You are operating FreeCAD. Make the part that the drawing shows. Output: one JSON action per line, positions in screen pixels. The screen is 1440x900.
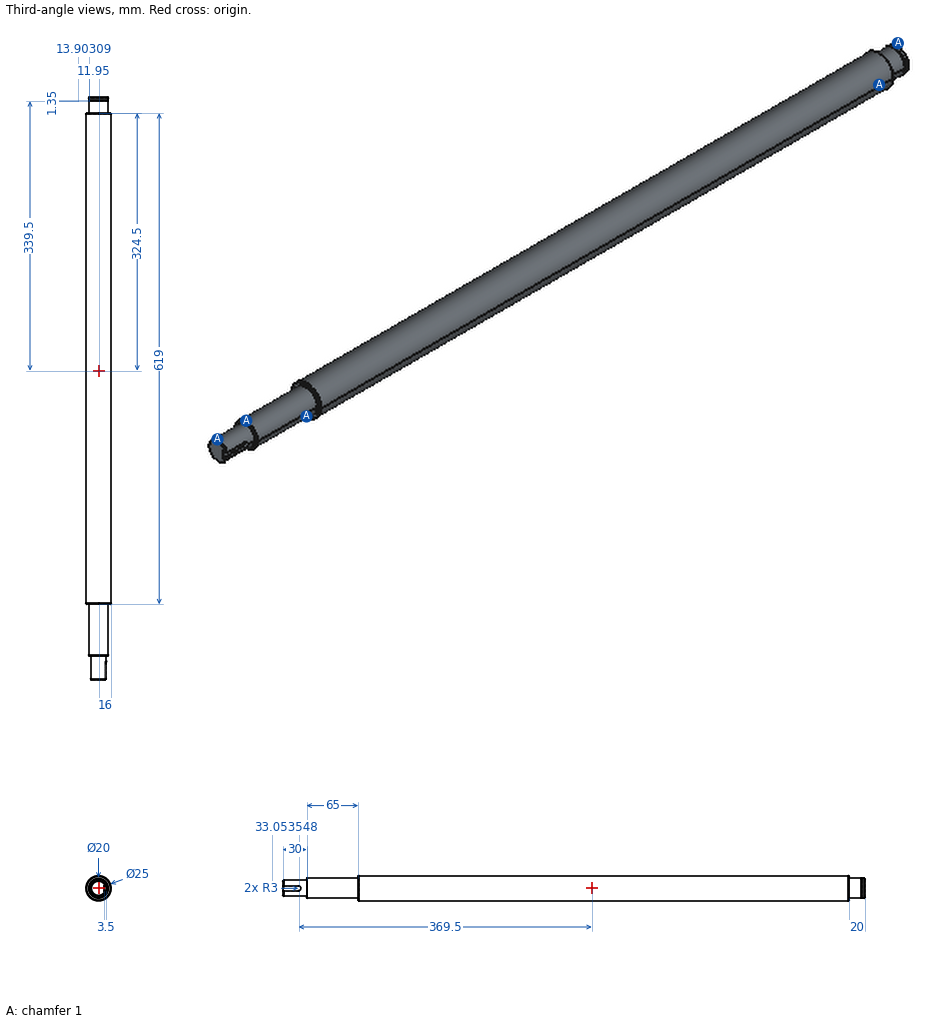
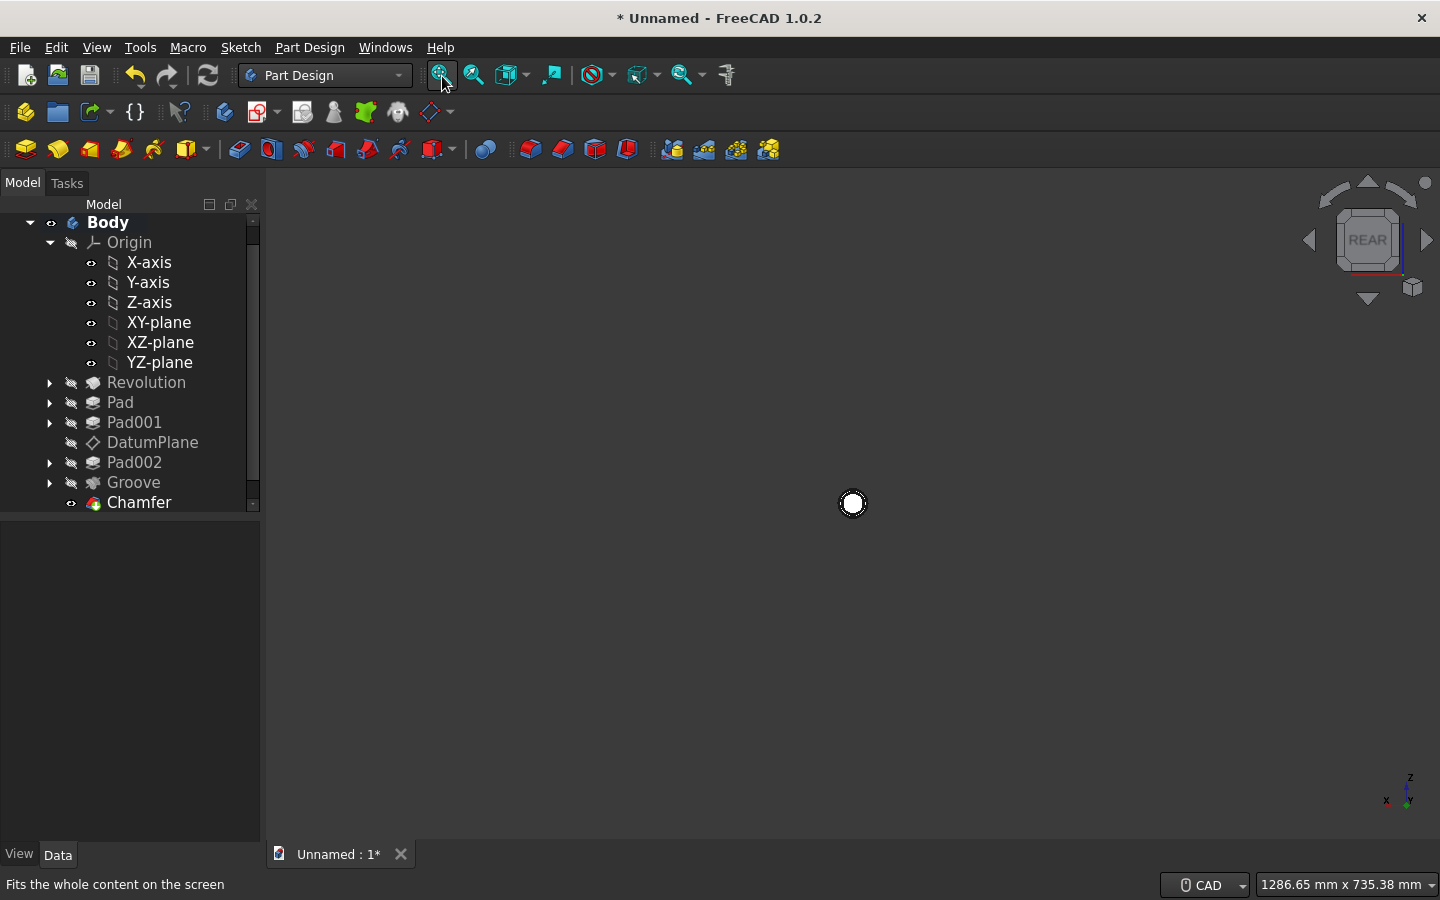
{"action": "left_click", "coordinate": [136, 363]}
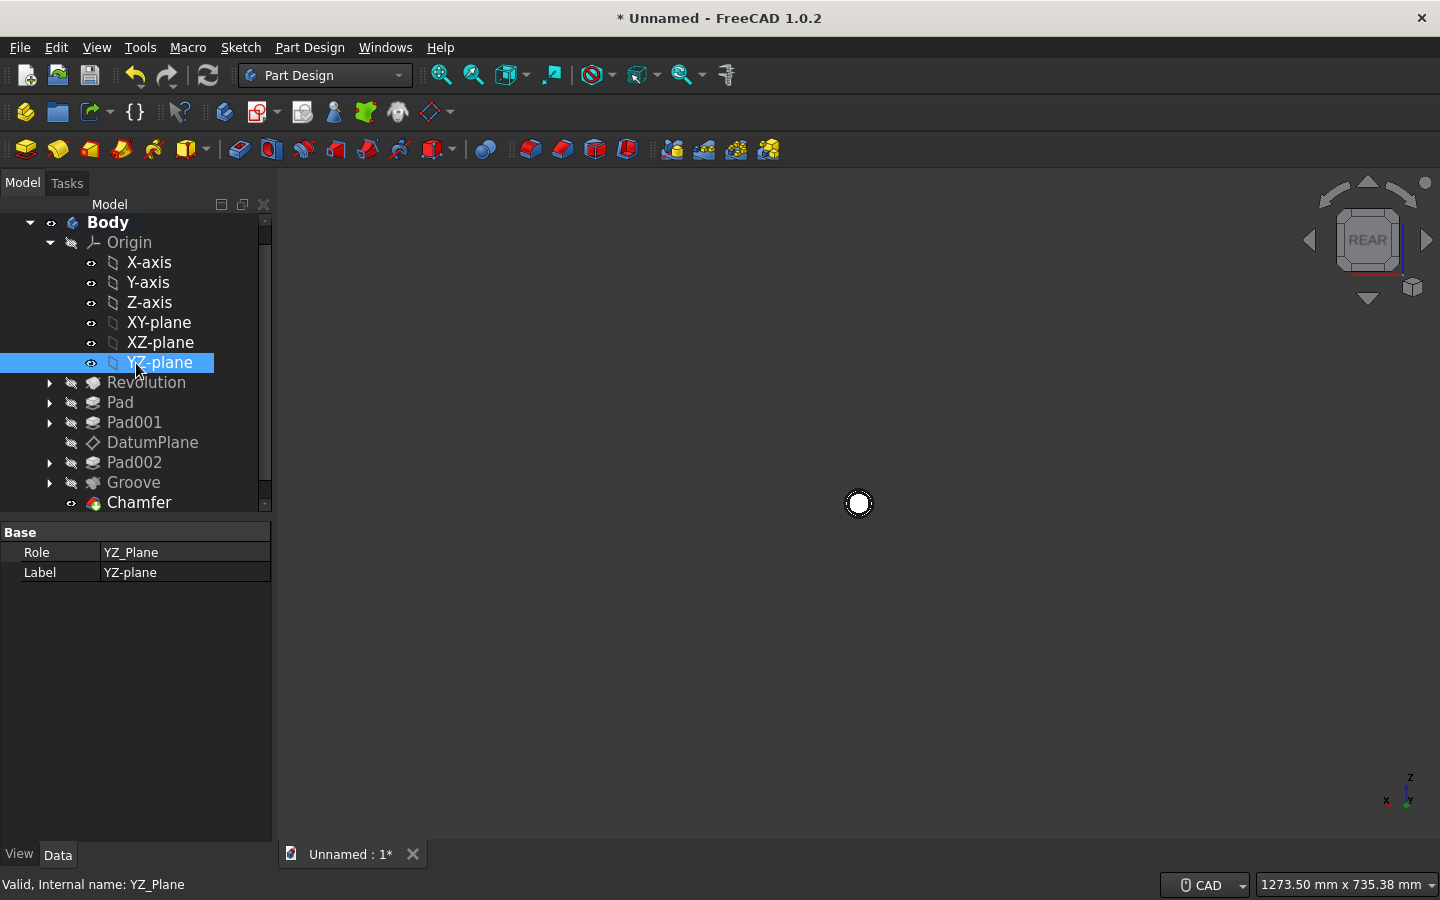
{"action": "left_click", "coordinate": [430, 112]}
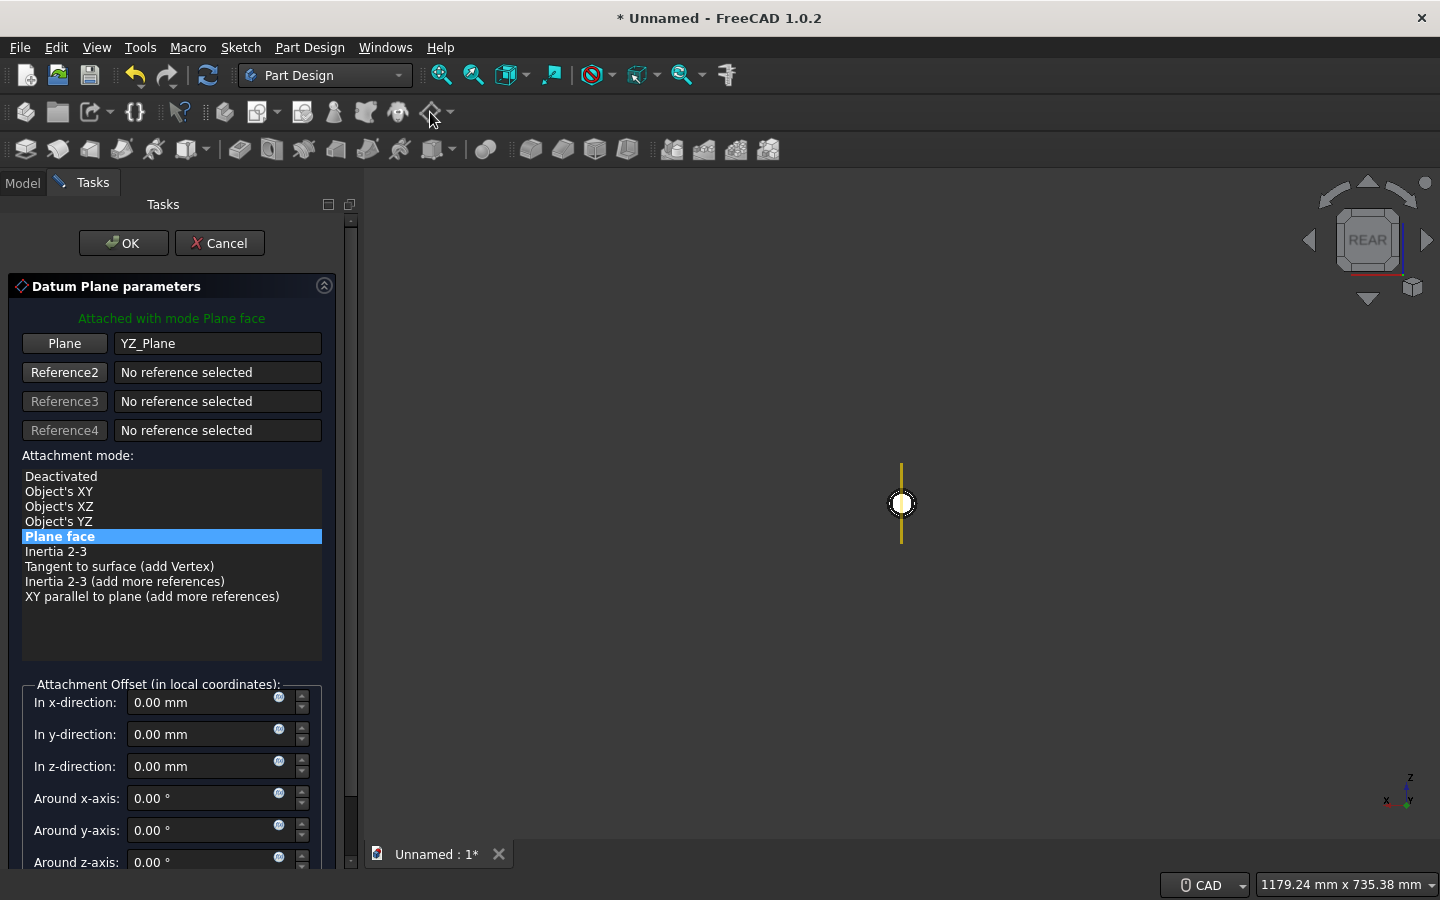
{"action": "triple_click", "coordinate": [210, 766]}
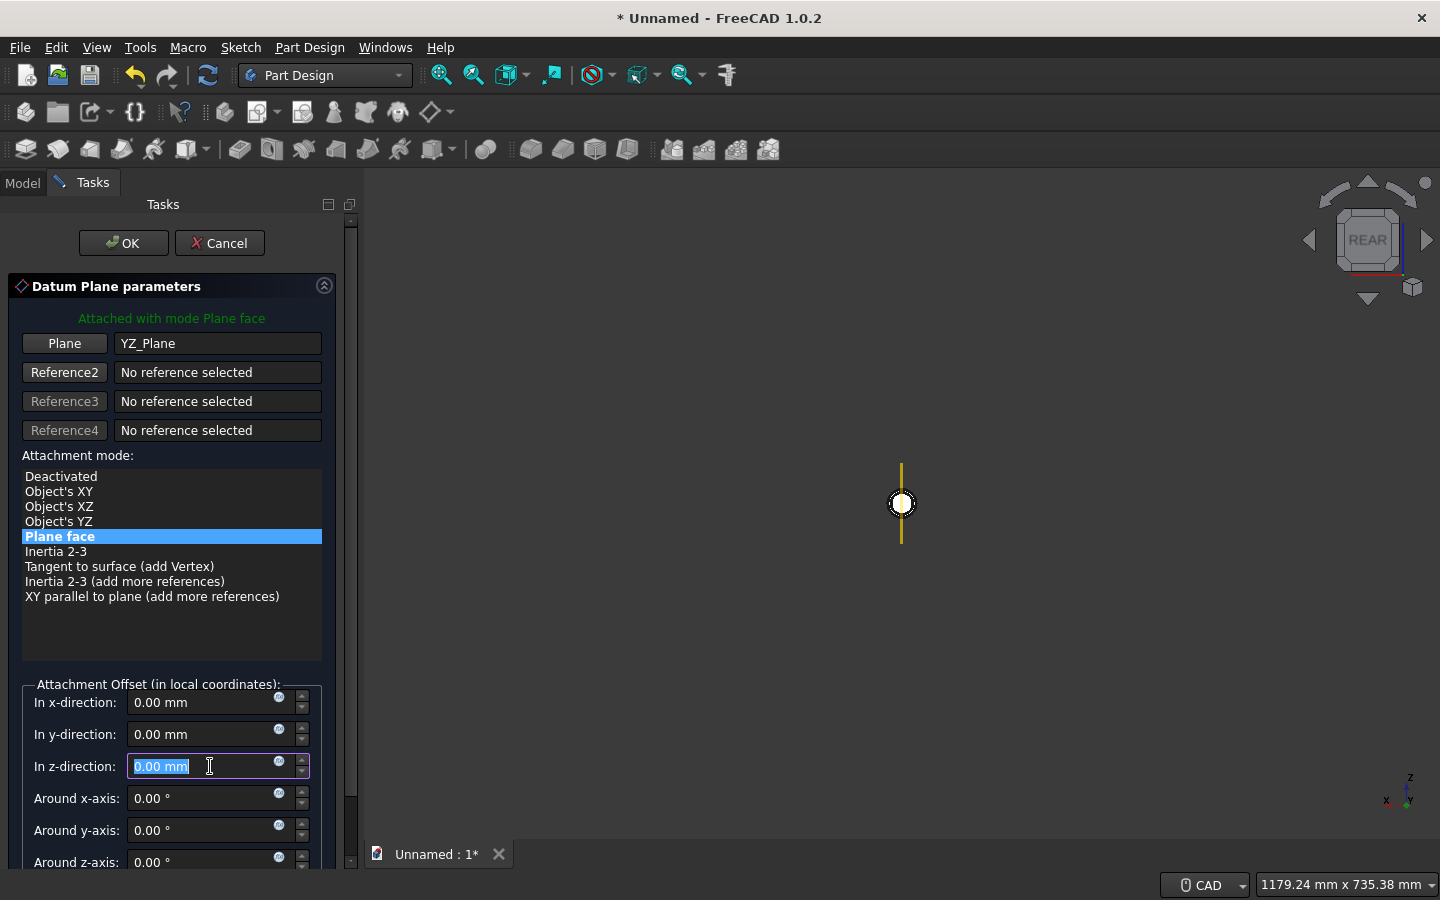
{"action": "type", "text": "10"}
{"action": "key", "text": "Tab"}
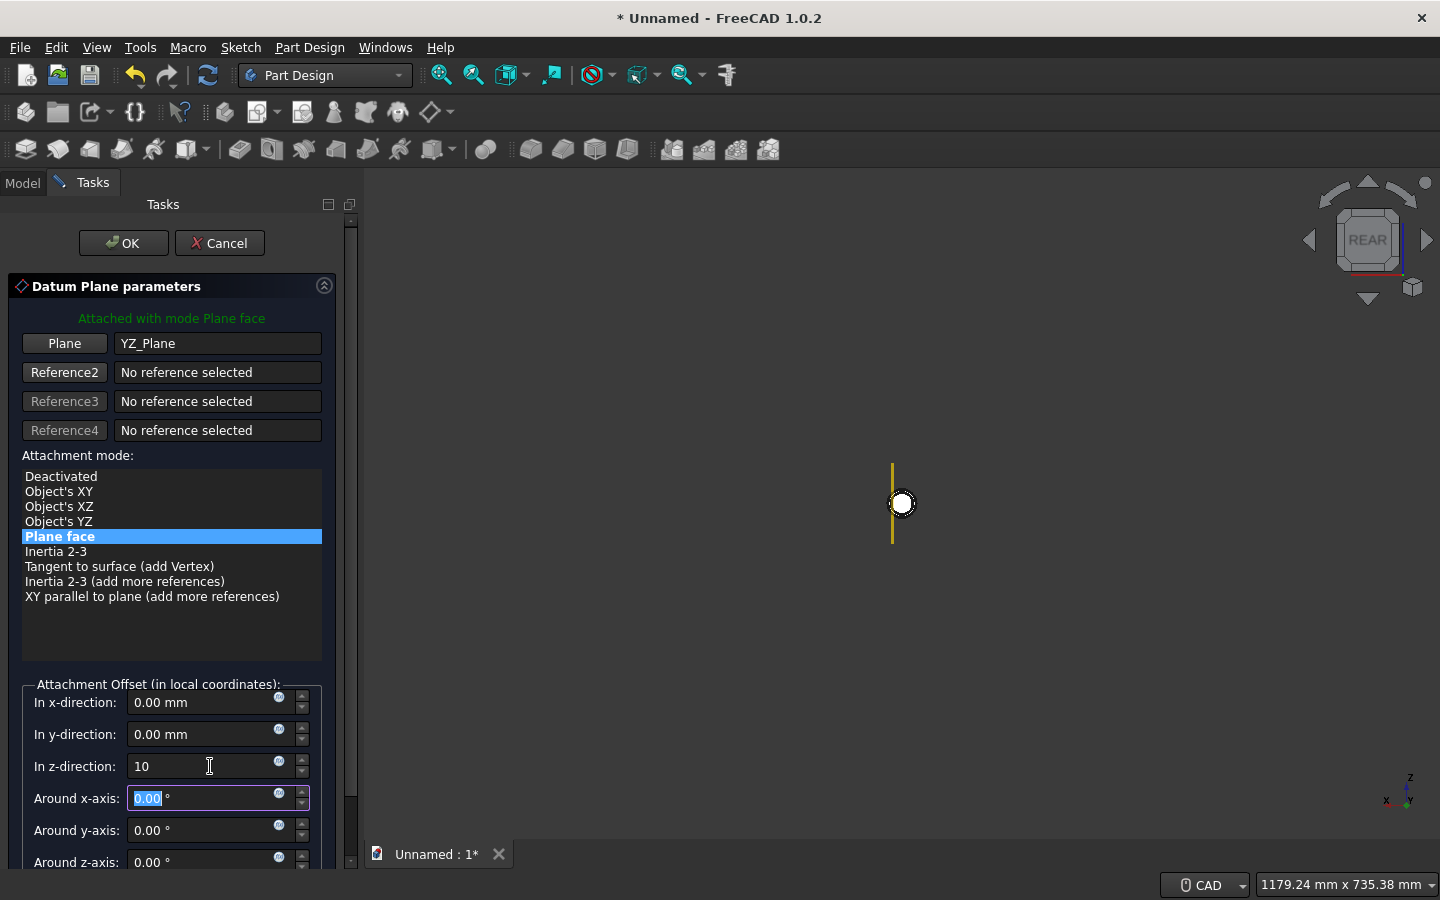
{"action": "left_click", "coordinate": [124, 243]}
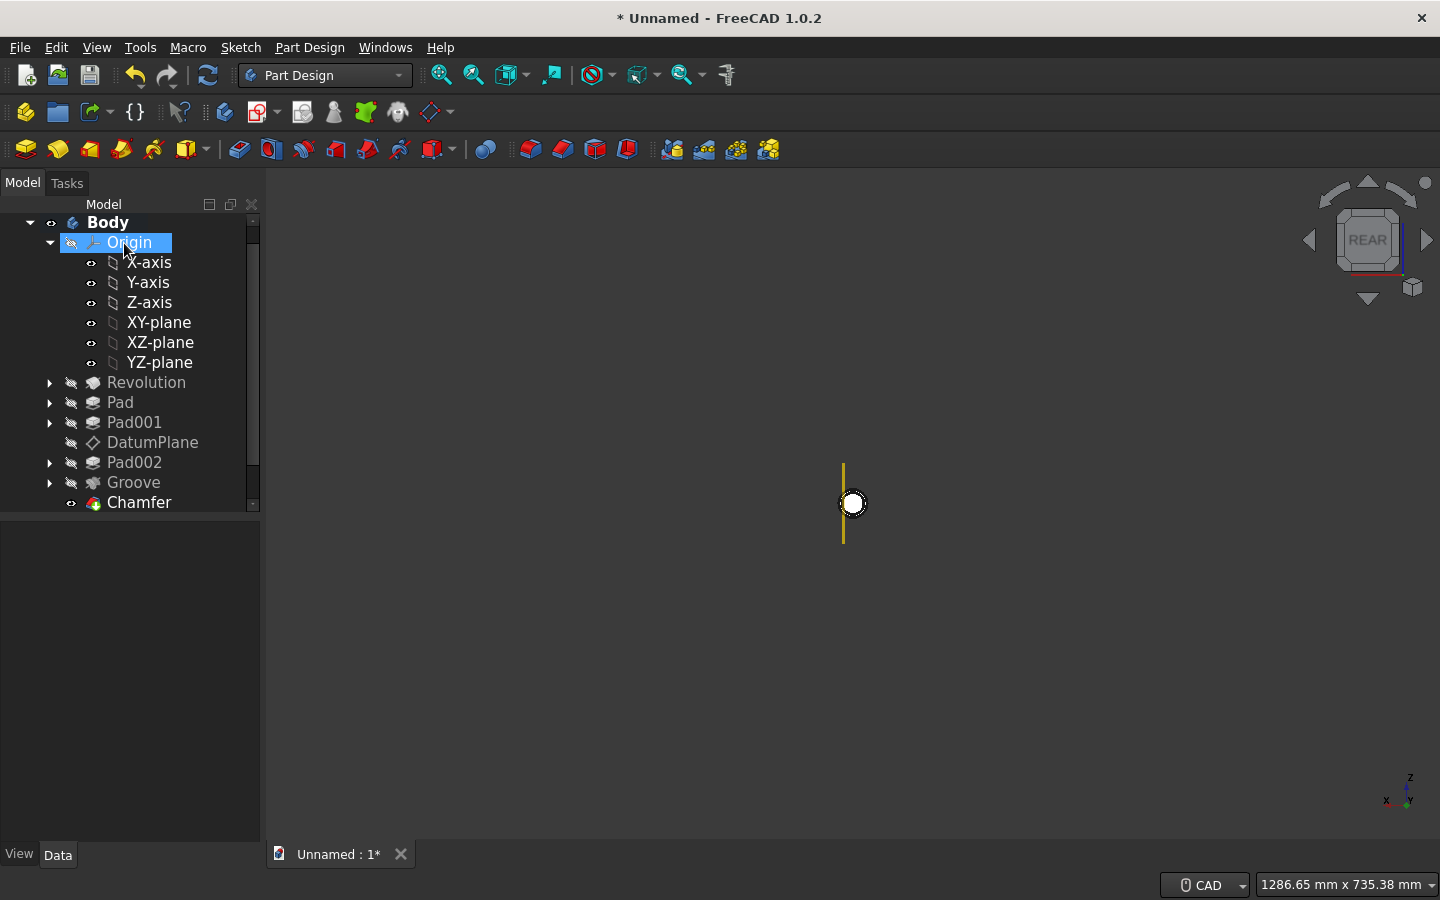
{"action": "scroll", "coordinate": [120, 358], "scroll_direction": "down", "scroll_amount": 3}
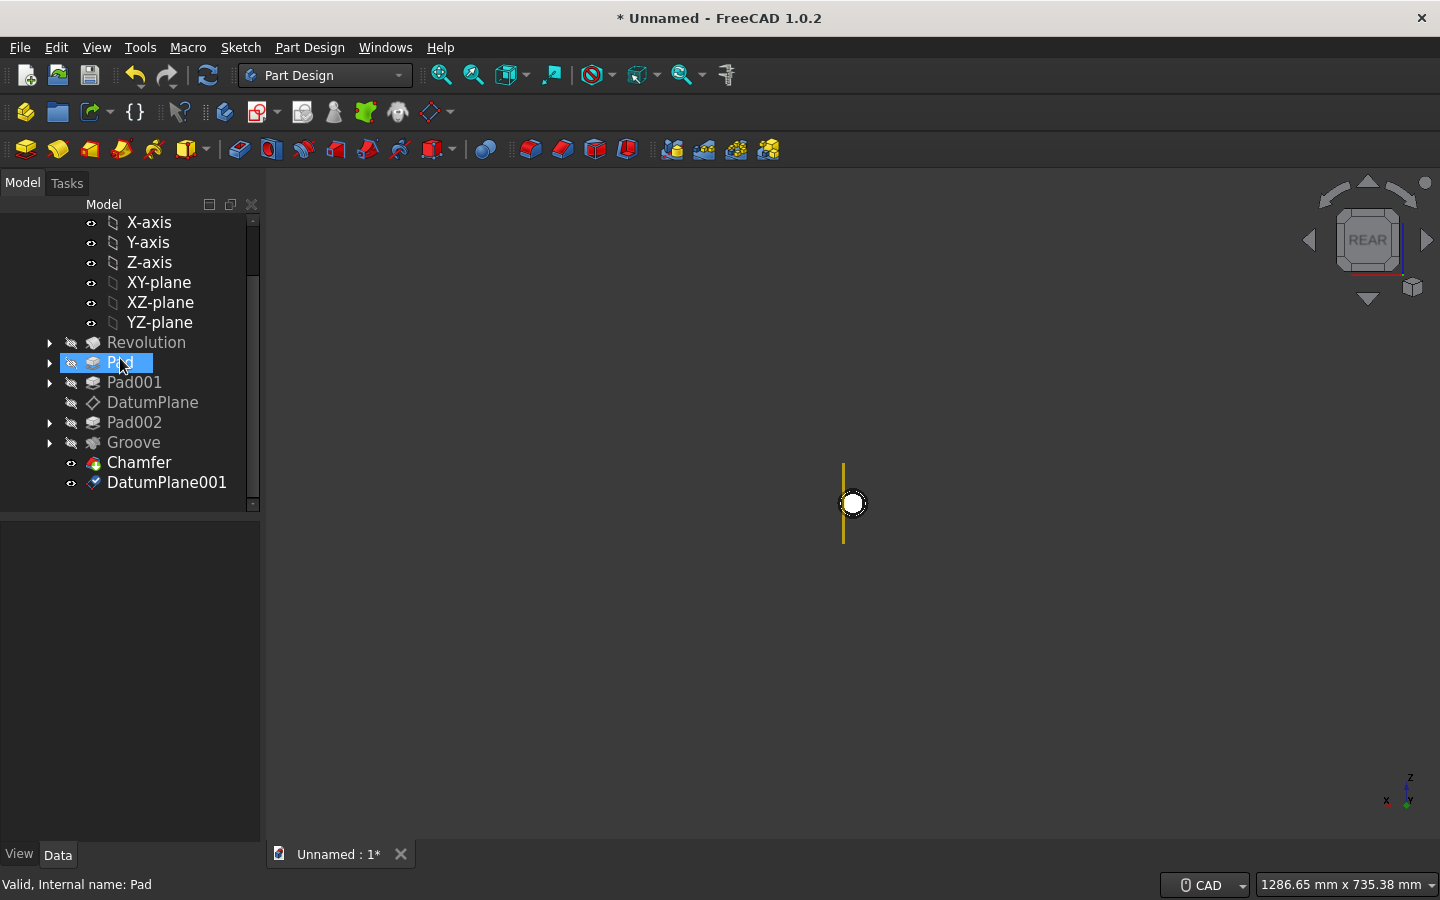
{"action": "left_click", "coordinate": [116, 483]}